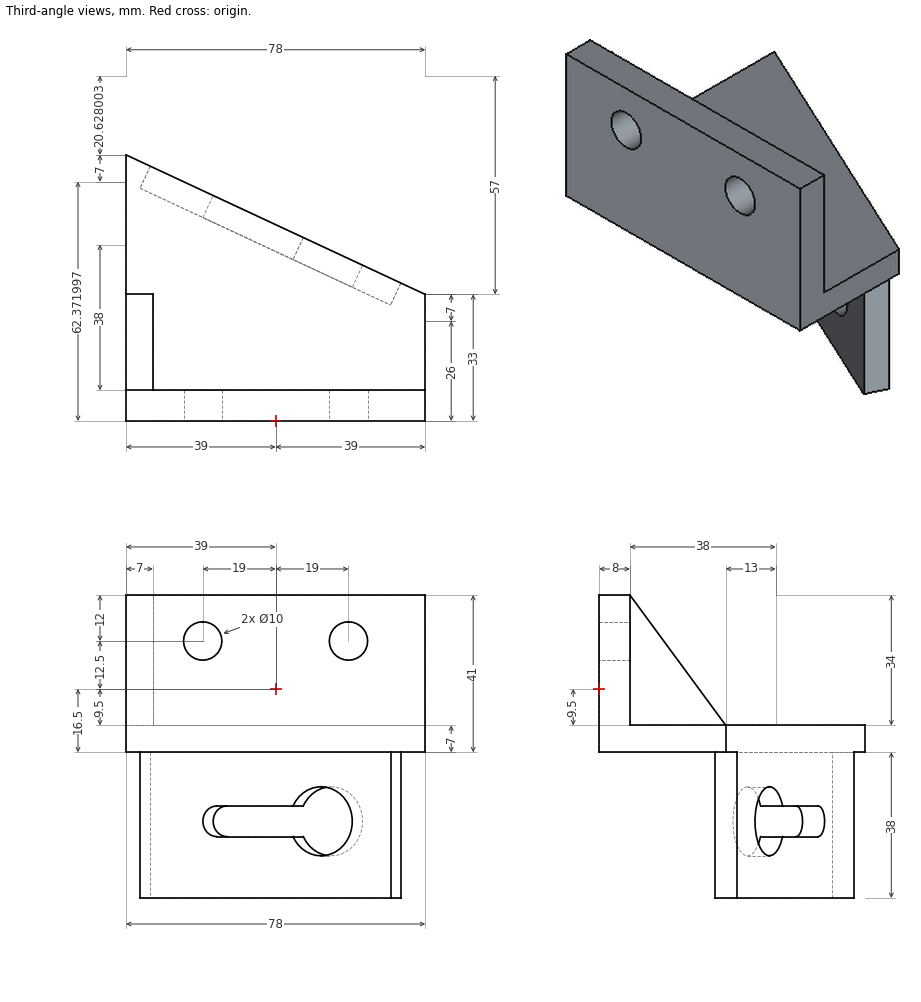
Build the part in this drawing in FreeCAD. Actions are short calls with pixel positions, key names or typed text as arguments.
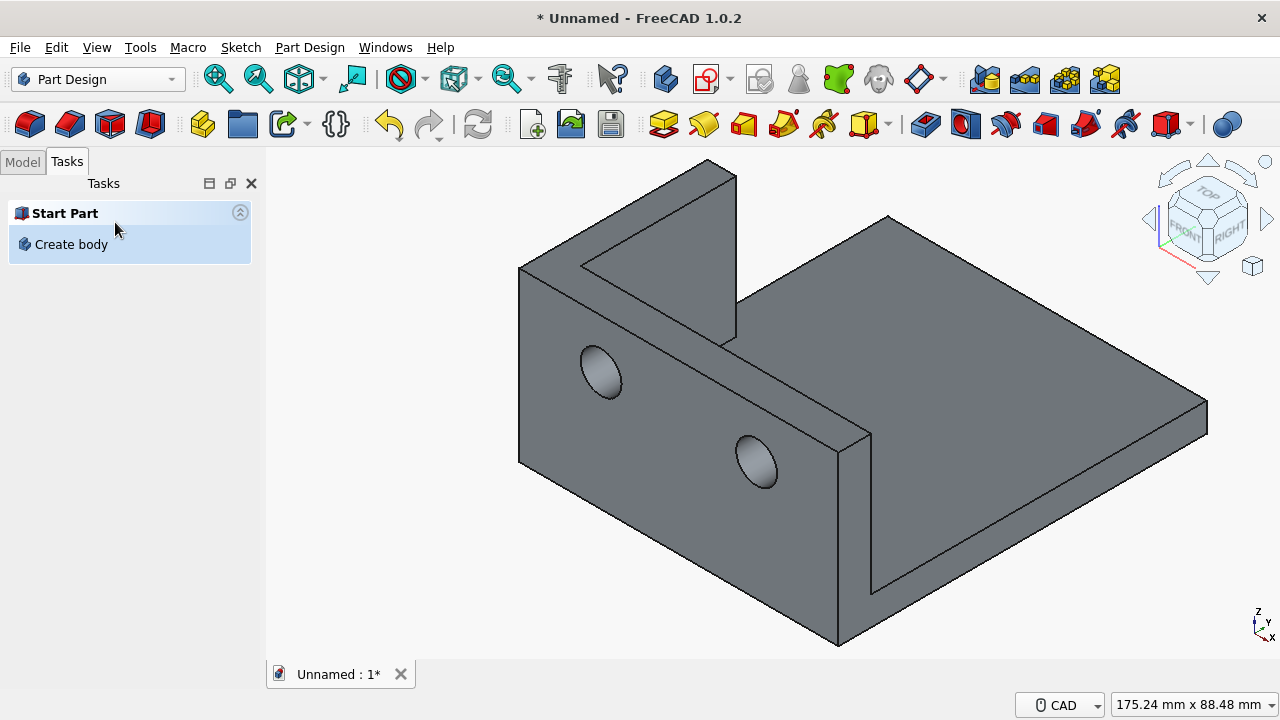
click(220, 80)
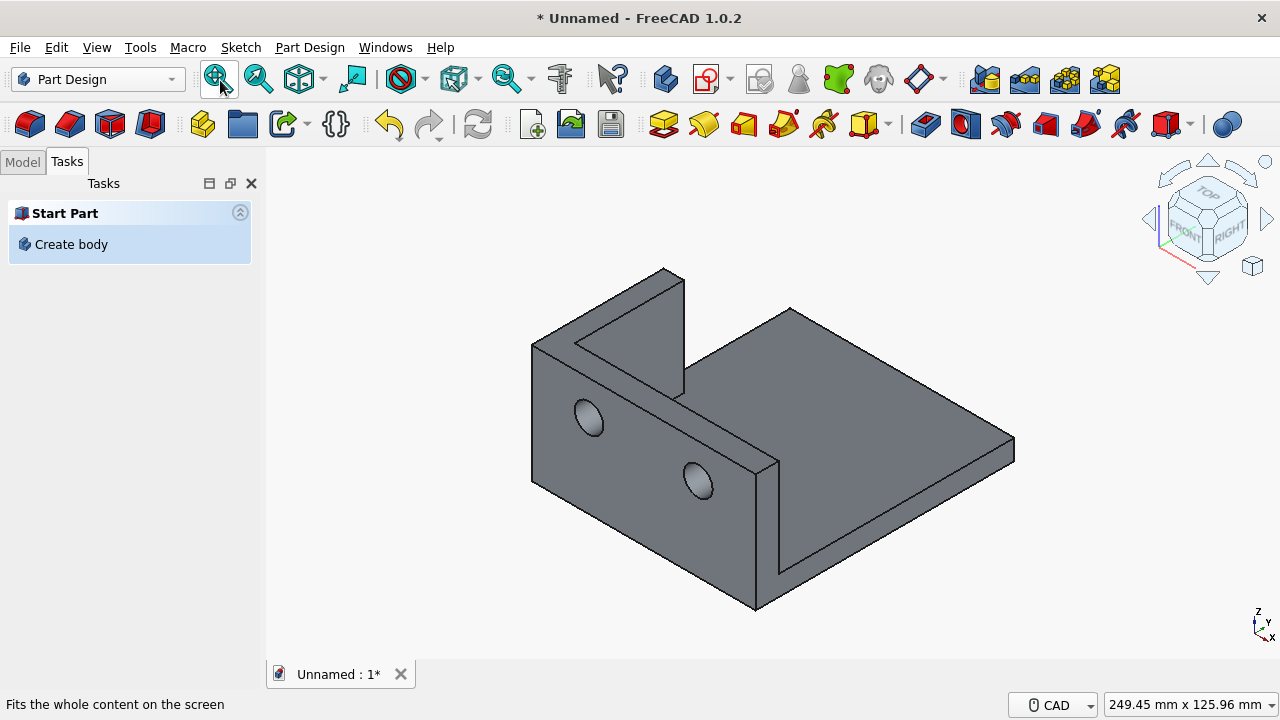
click(645, 358)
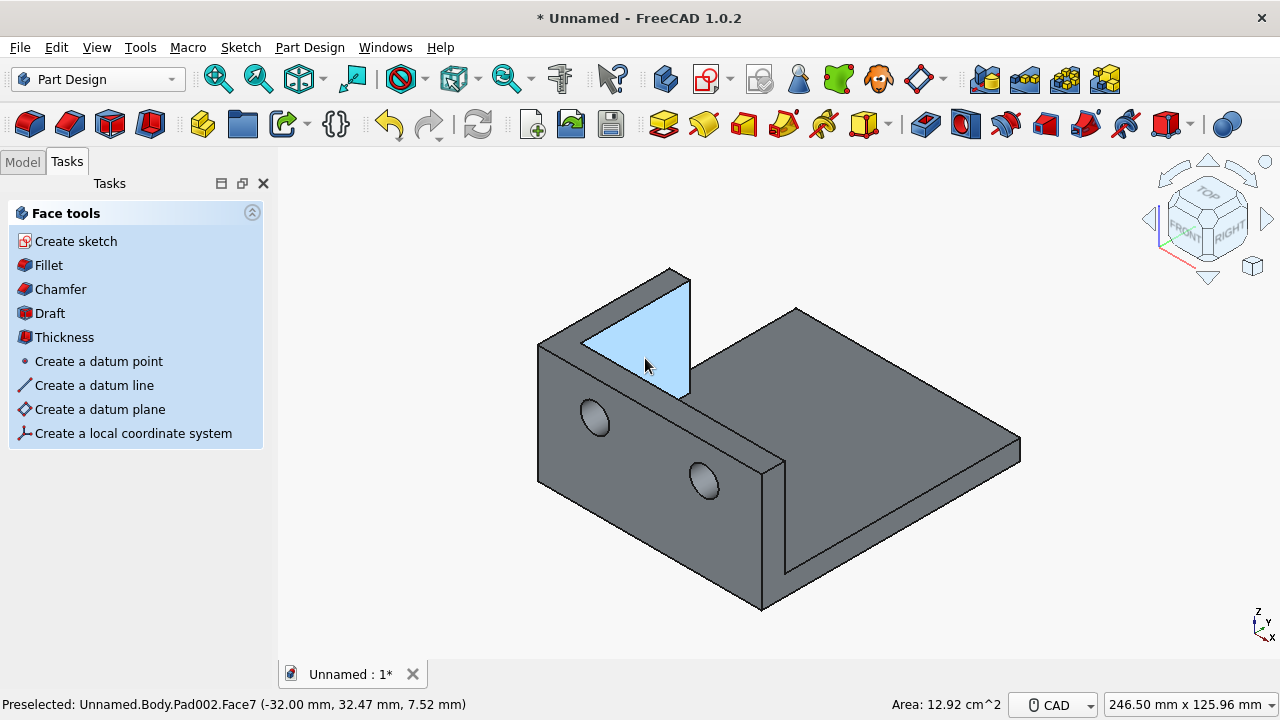
click(706, 80)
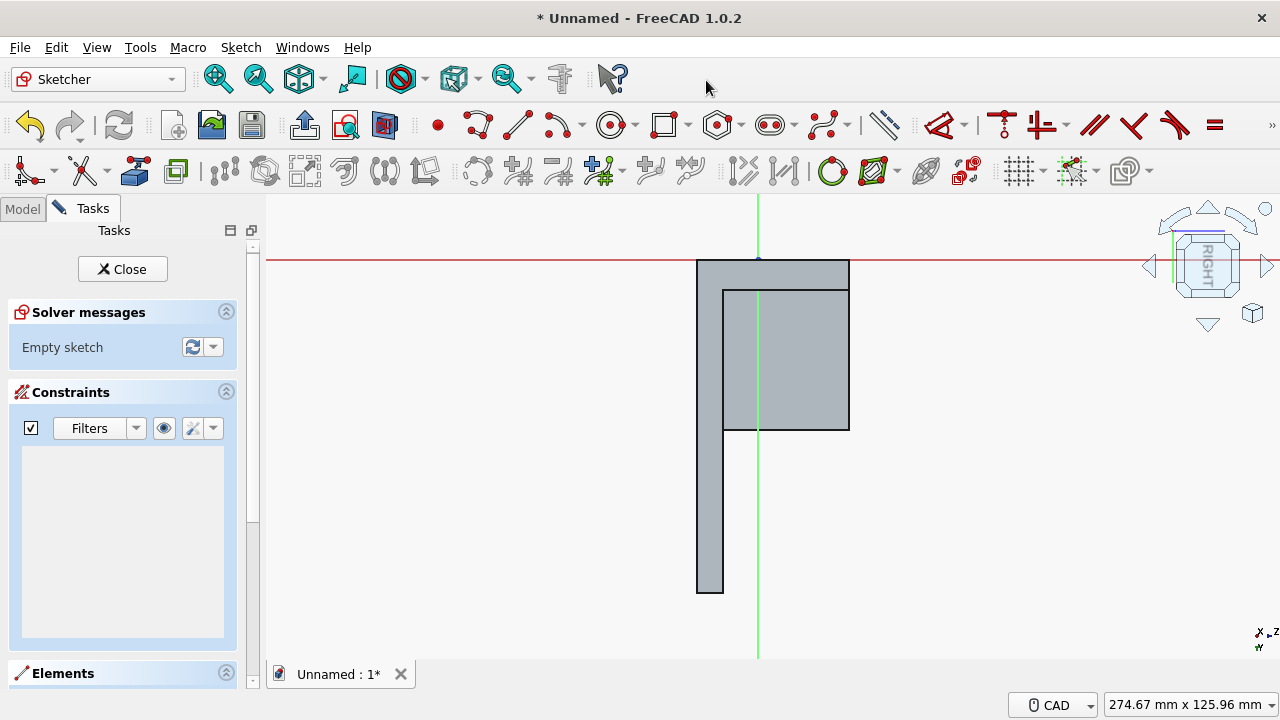
scroll(885, 246, up, 3)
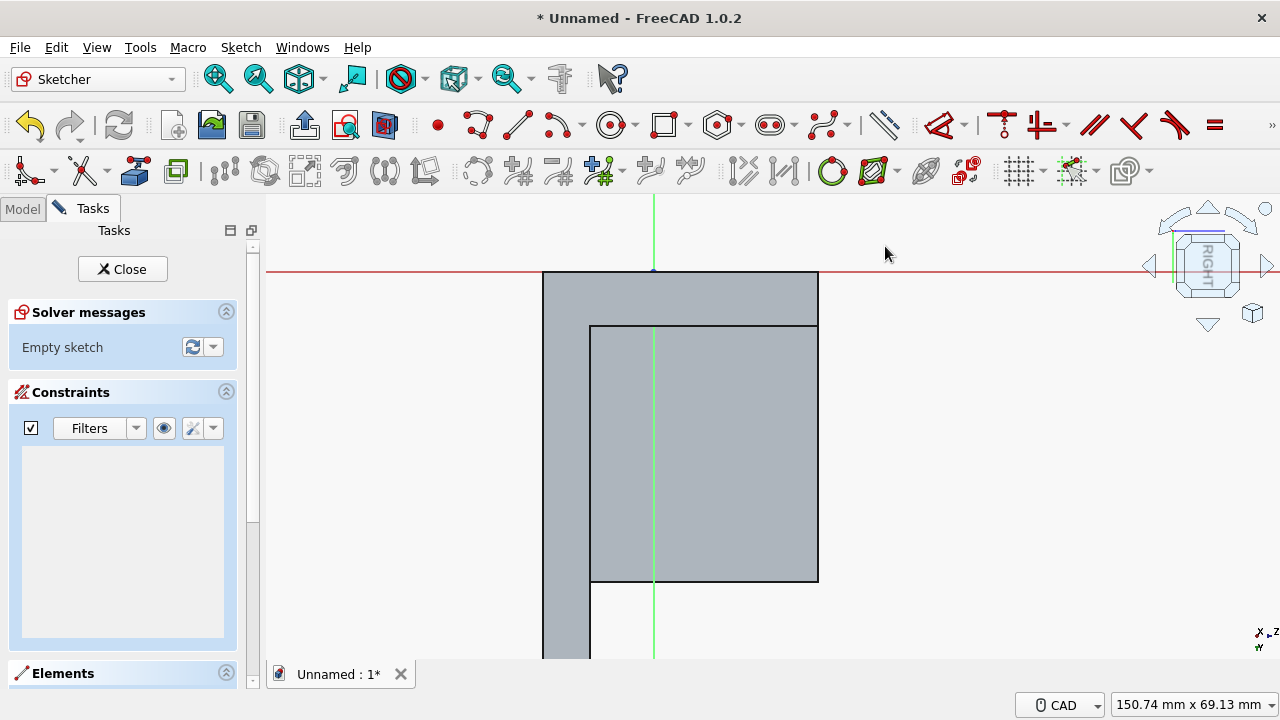
click(478, 126)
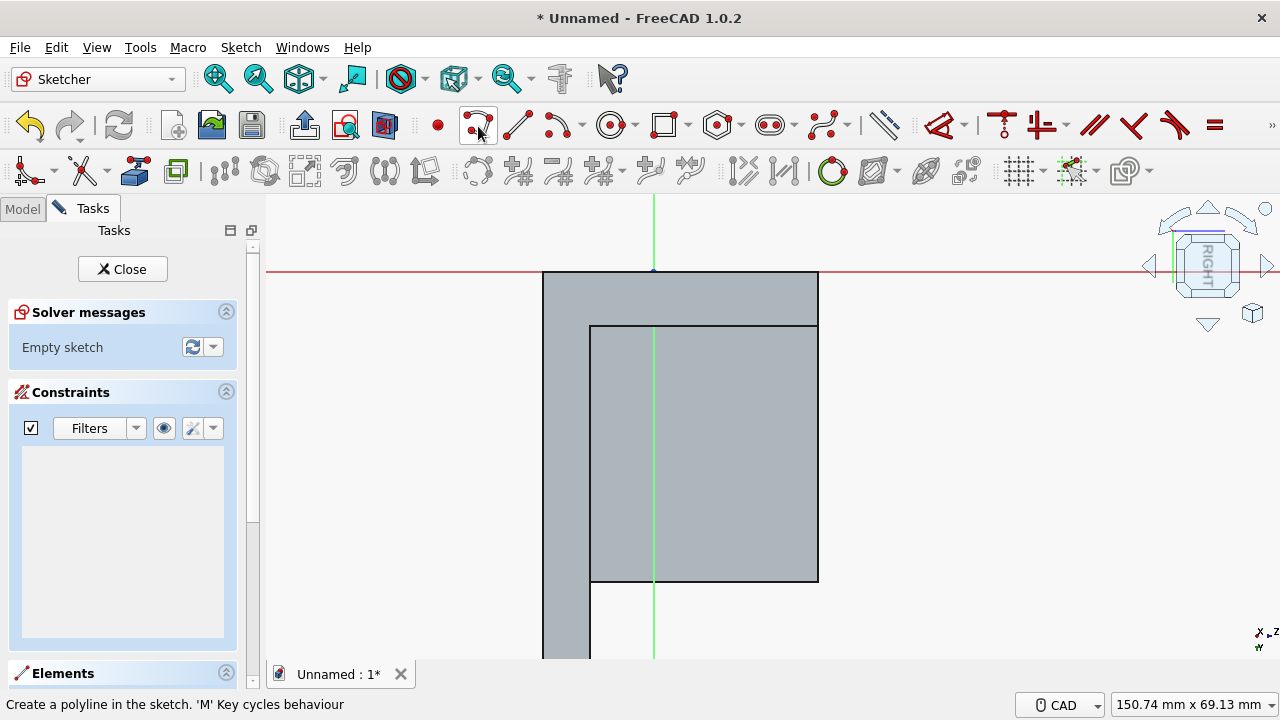
click(818, 326)
click(590, 494)
click(590, 582)
click(818, 582)
click(818, 327)
key(Escape)
key(Escape)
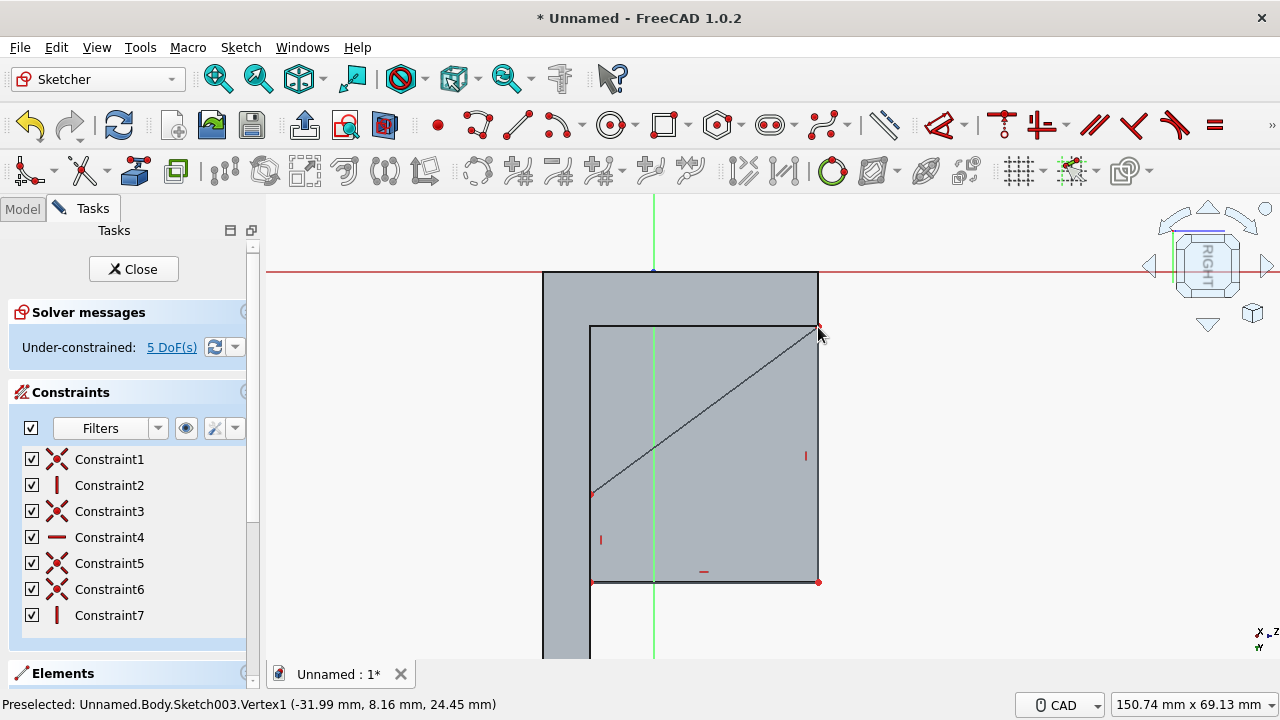
click(940, 126)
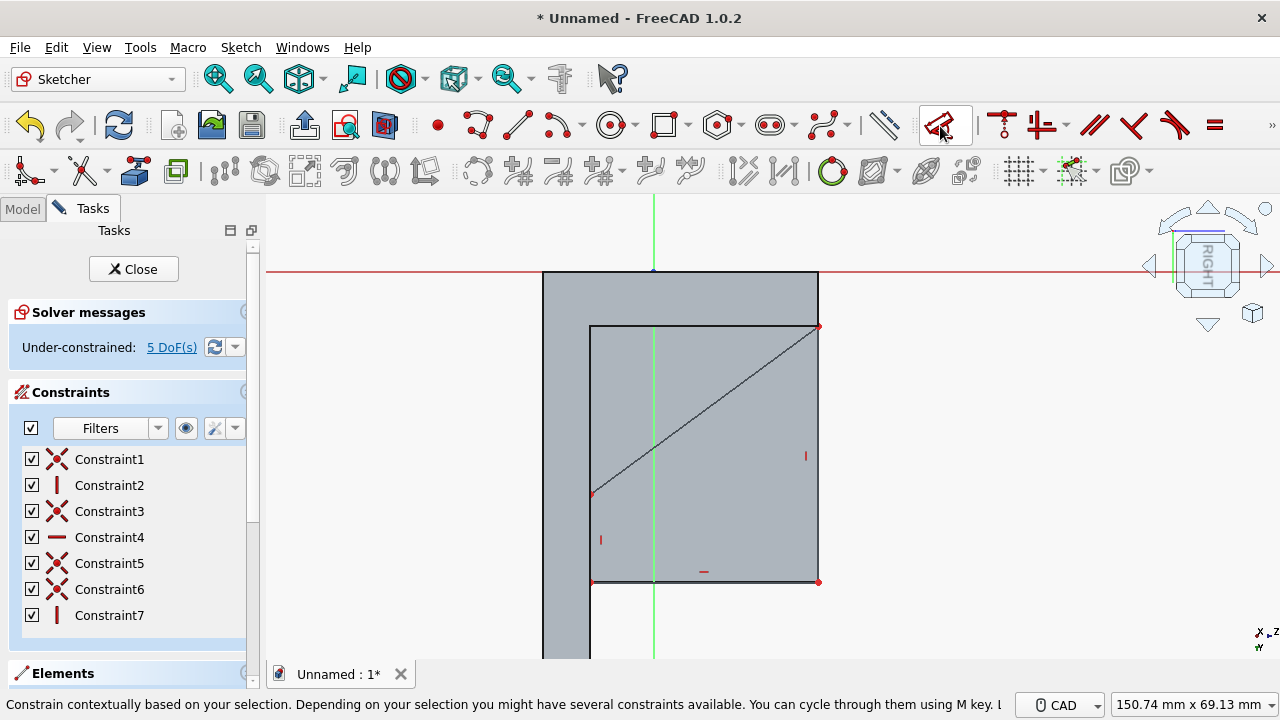
click(590, 521)
click(556, 539)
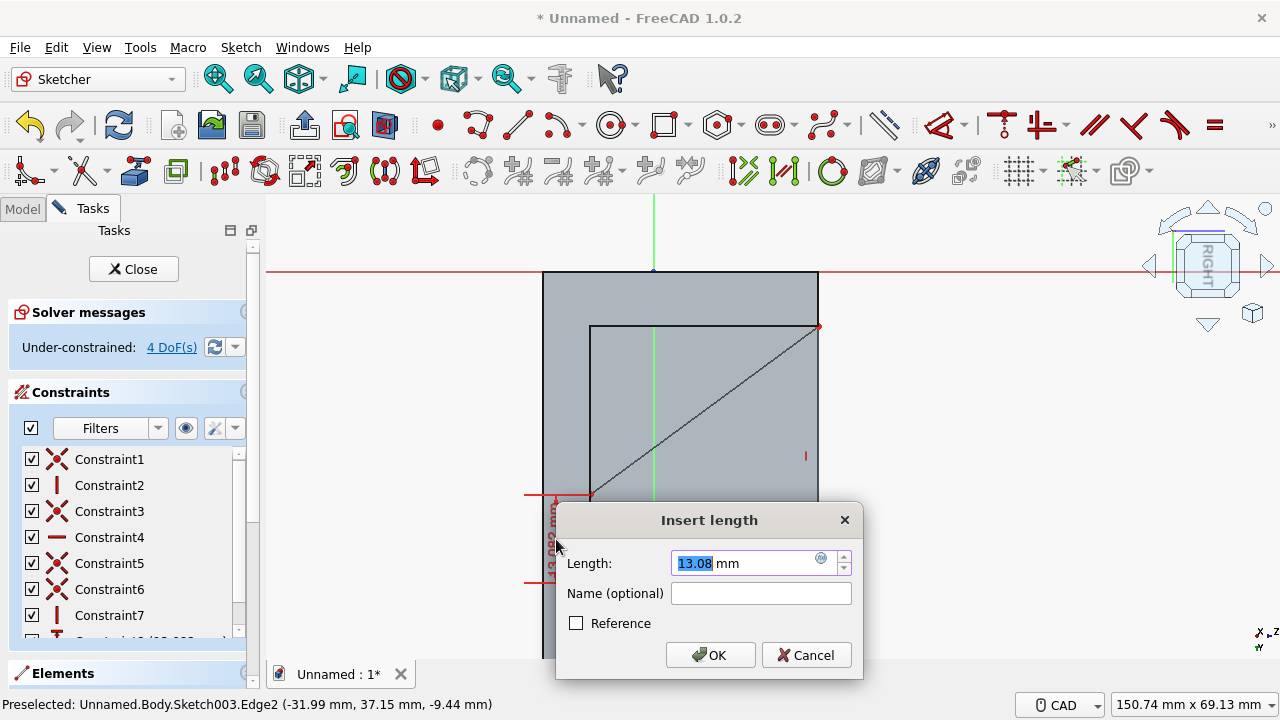
text(13)
key(Return)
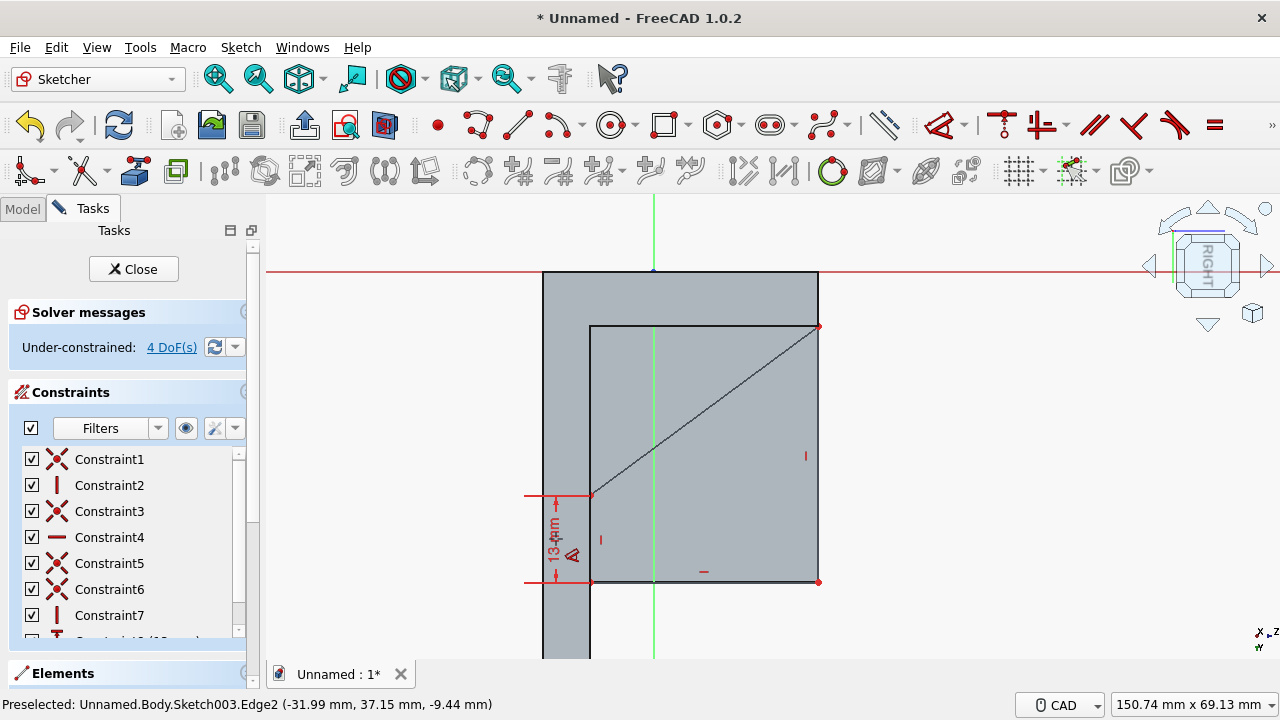
click(750, 583)
click(704, 617)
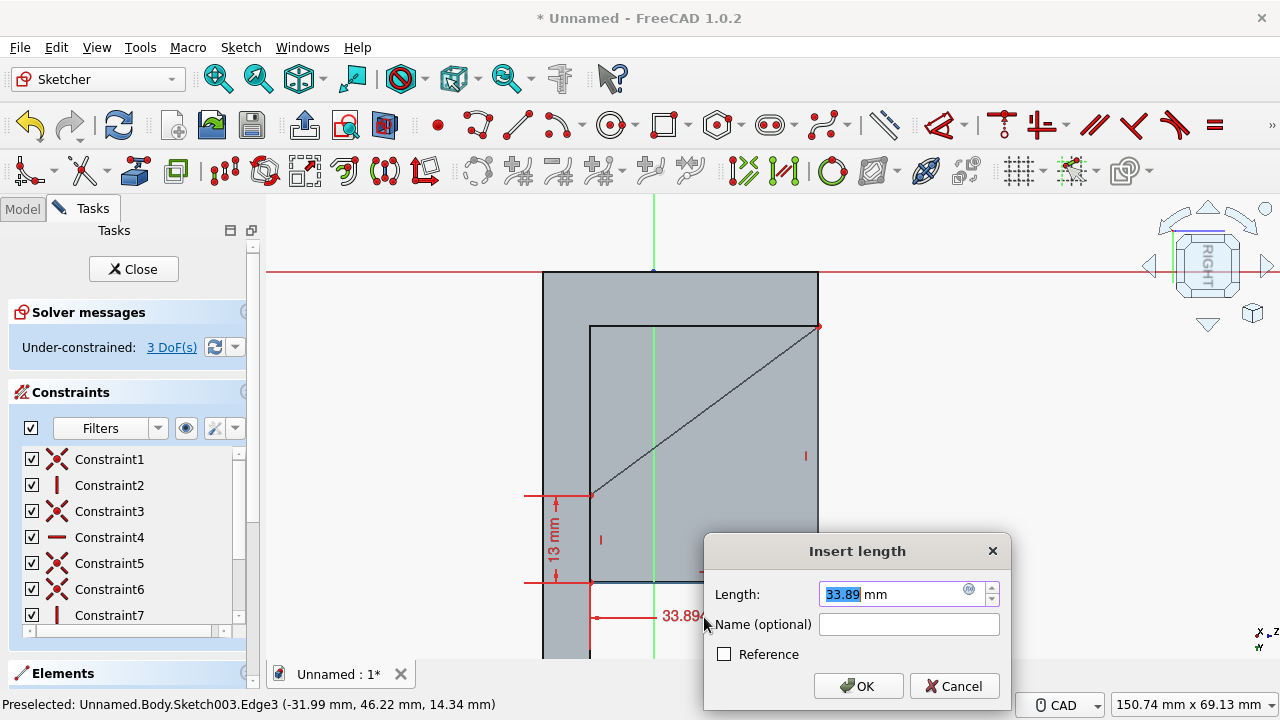
text(34)
key(Return)